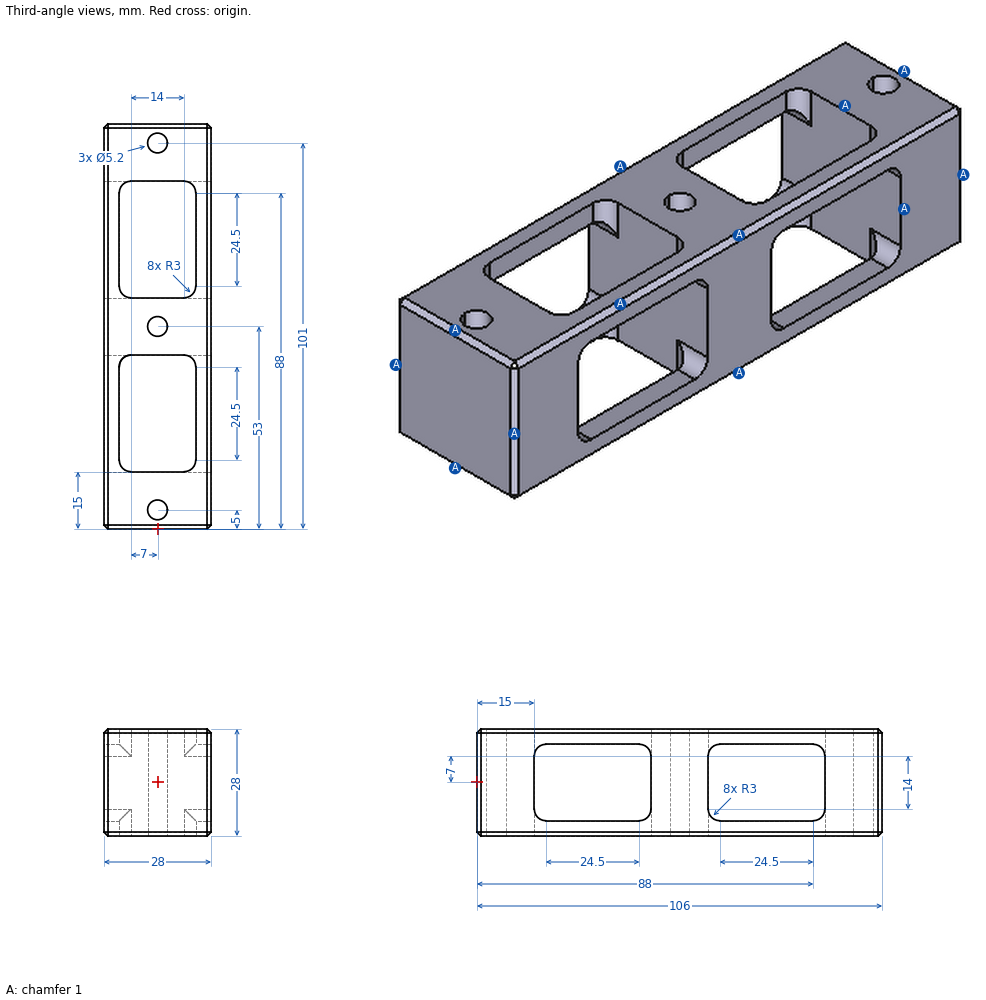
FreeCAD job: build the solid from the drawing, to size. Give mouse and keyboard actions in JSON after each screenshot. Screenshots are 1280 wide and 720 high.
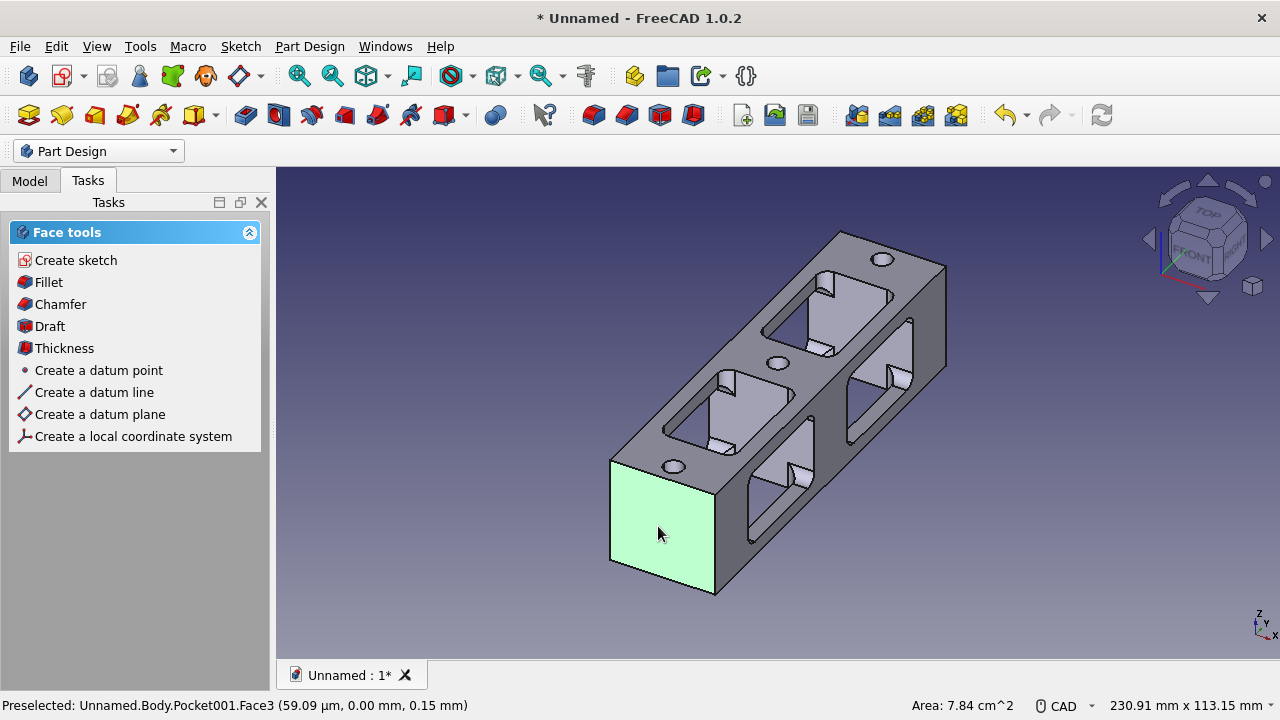
{"action": "left_click", "coordinate": [831, 380], "text": "ctrl"}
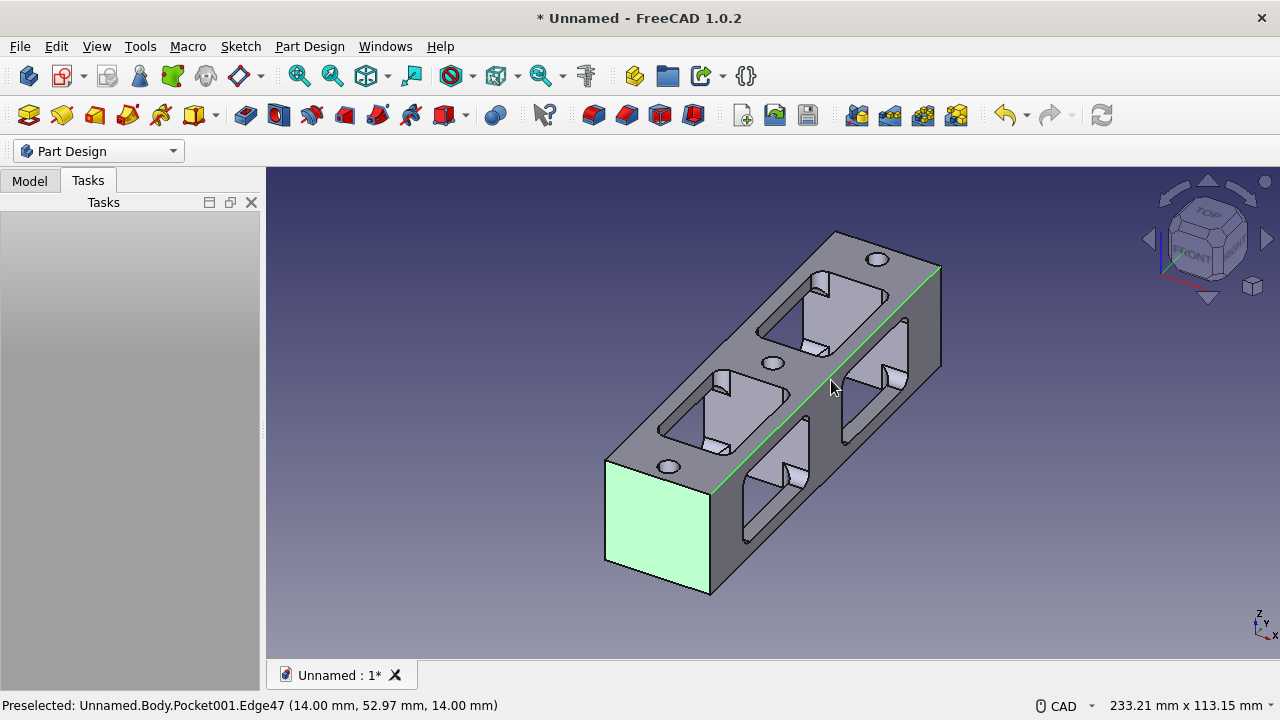
{"action": "key", "text": "0"}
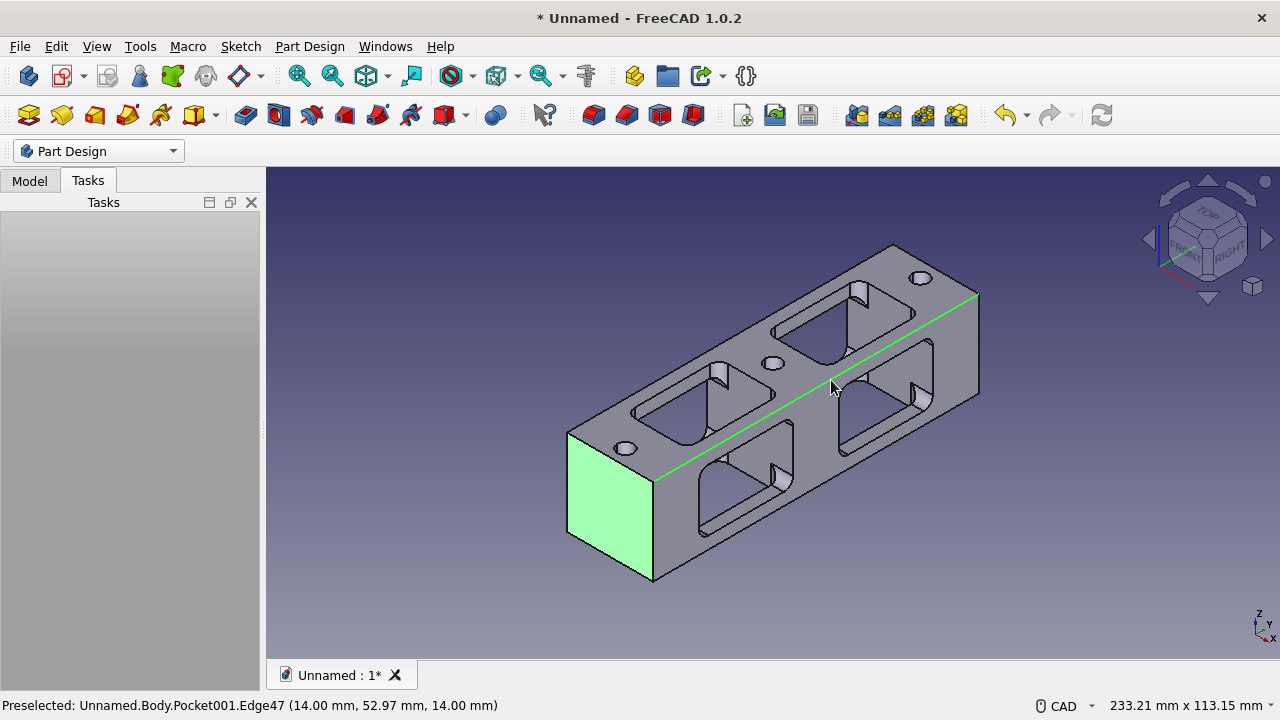
{"action": "key", "text": "2"}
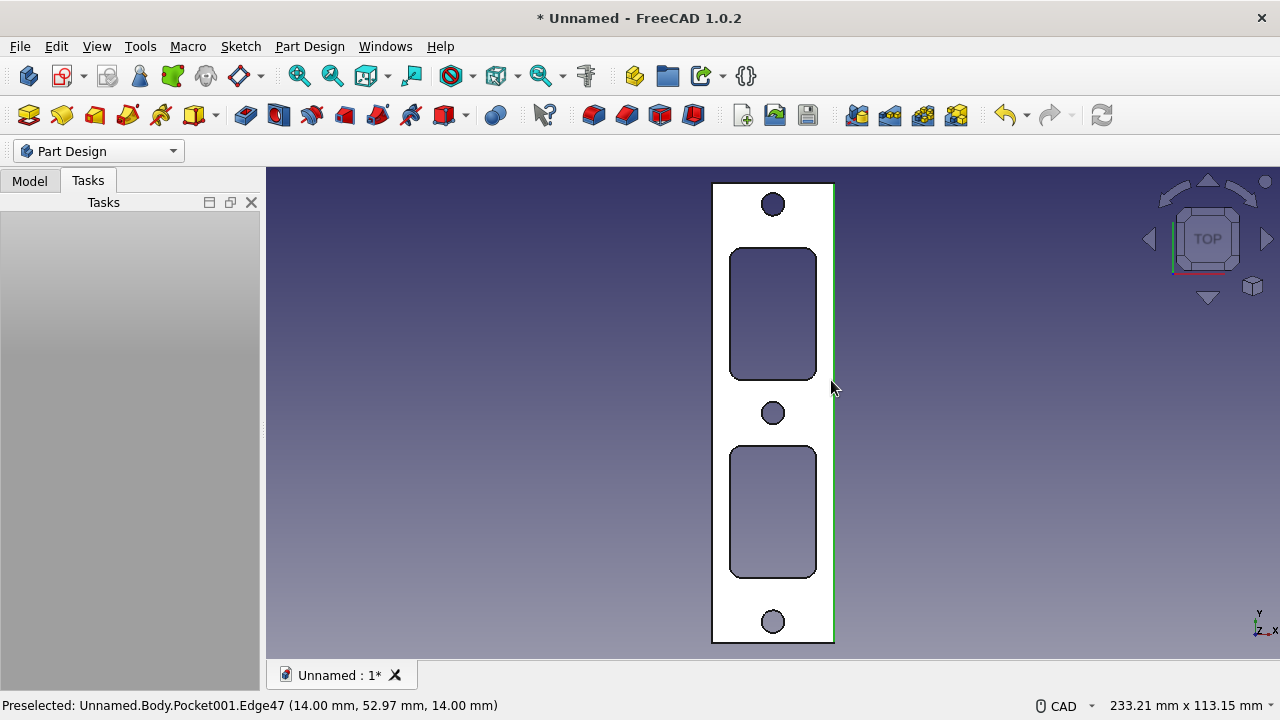
{"action": "left_click", "coordinate": [712, 412], "text": "ctrl"}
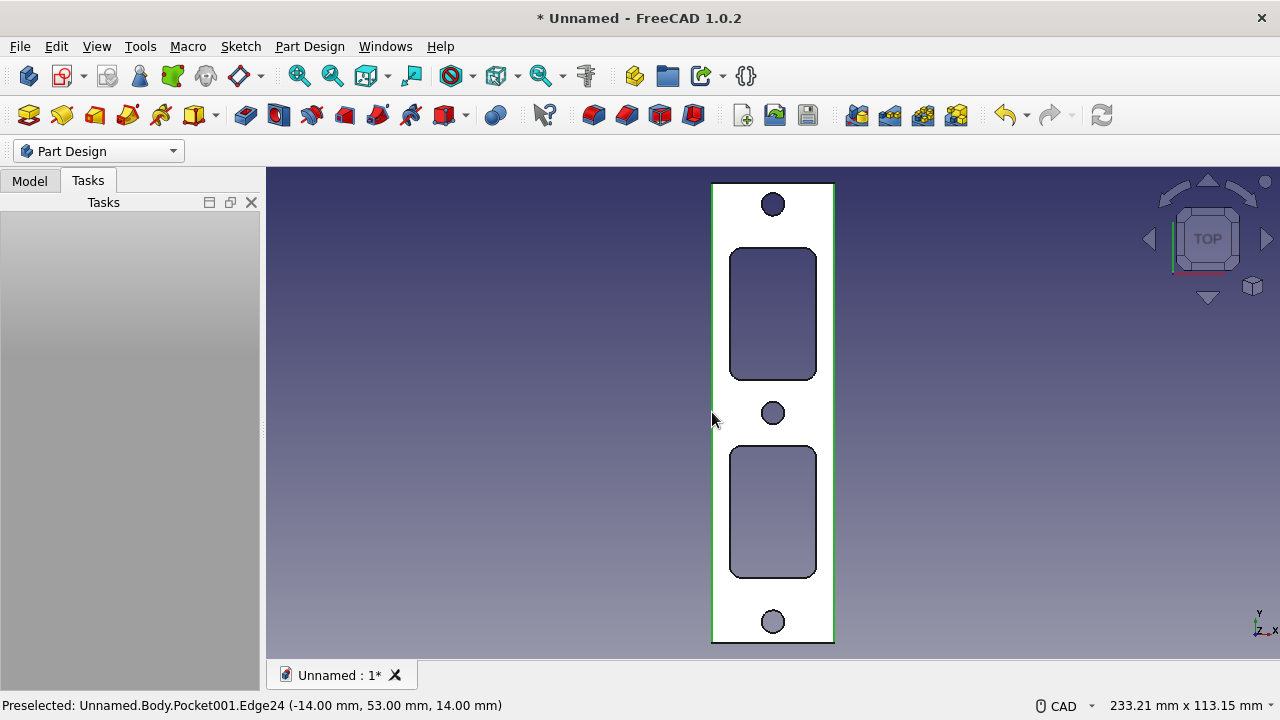
{"action": "key", "text": "1"}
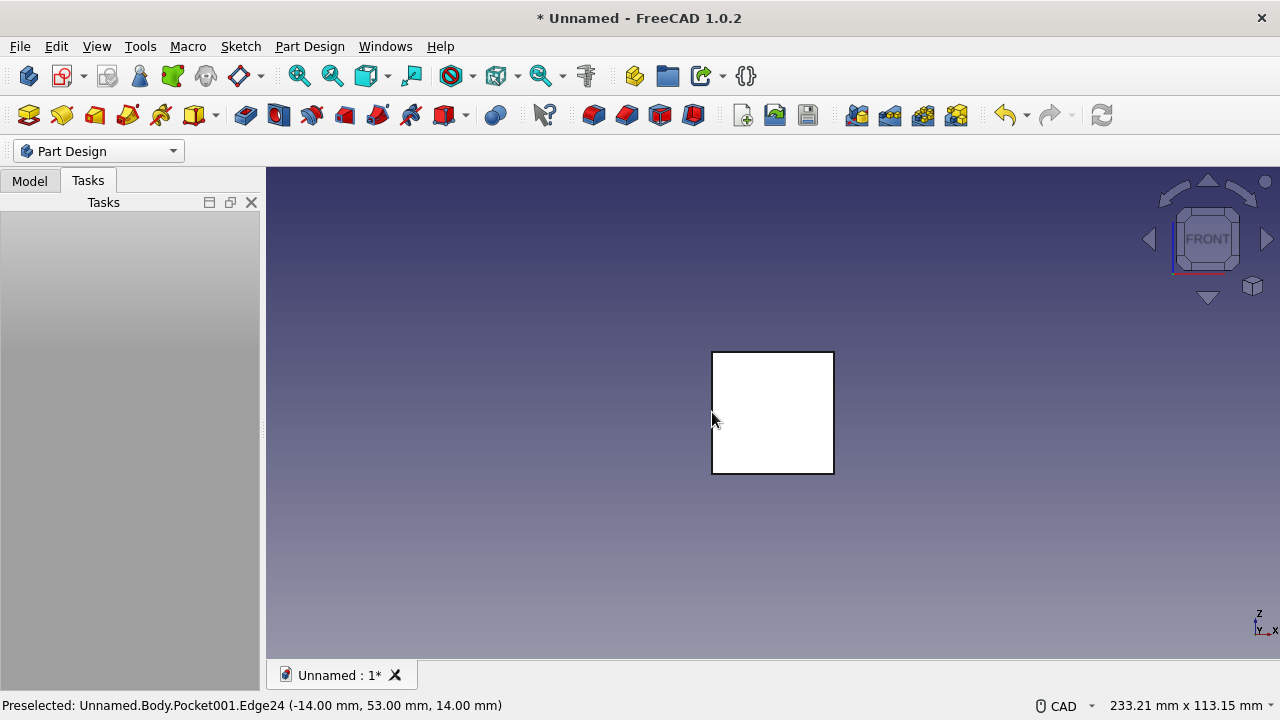
{"action": "left_click", "coordinate": [300, 76]}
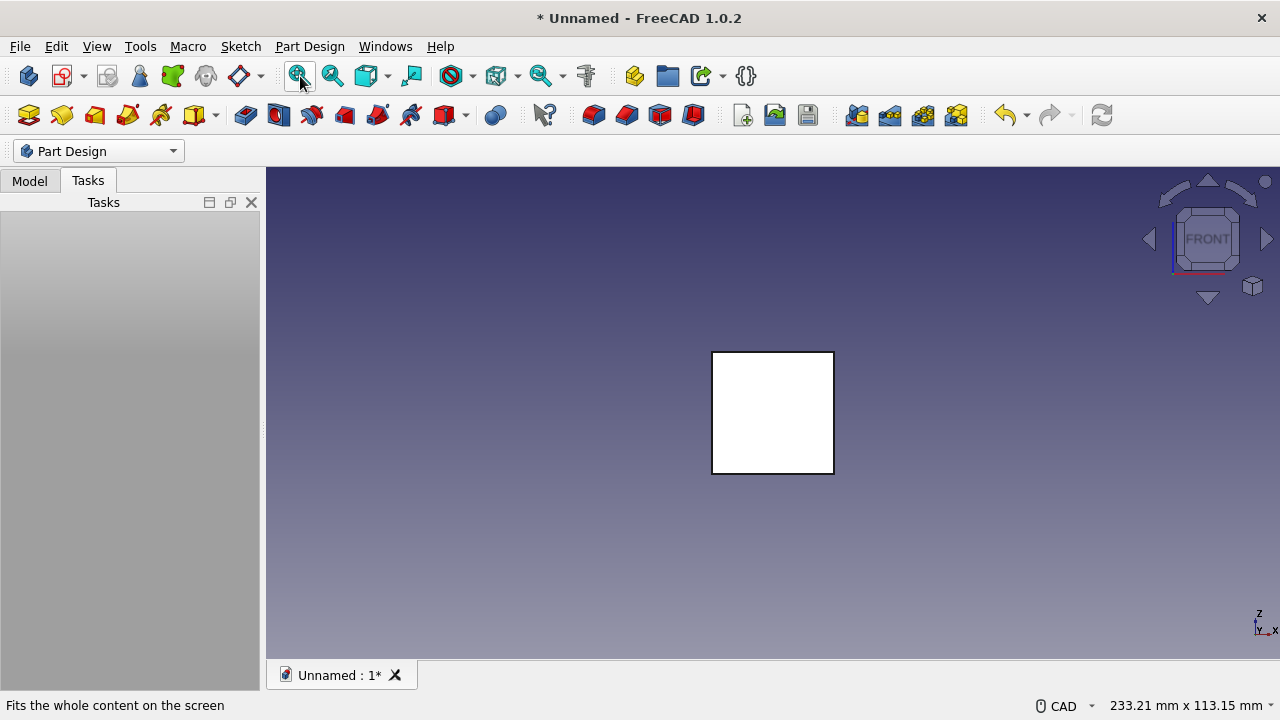
{"action": "key", "text": "3"}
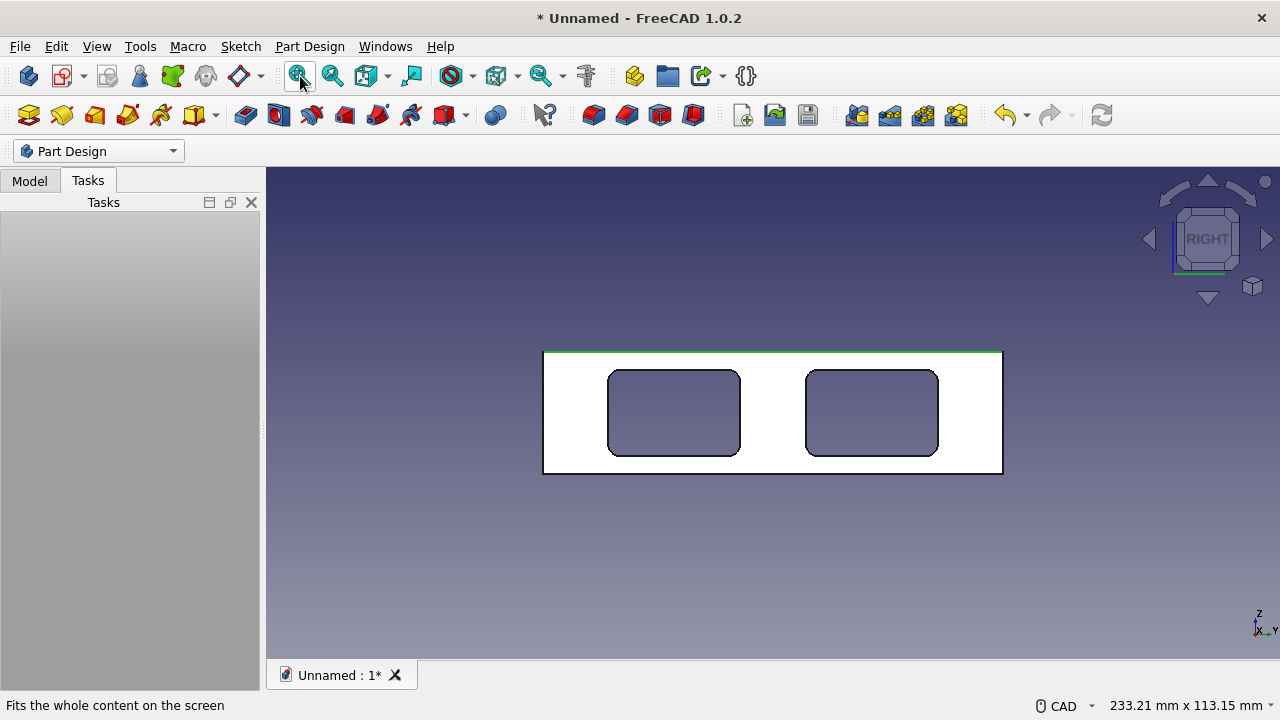
{"action": "left_click", "coordinate": [773, 473], "text": "ctrl"}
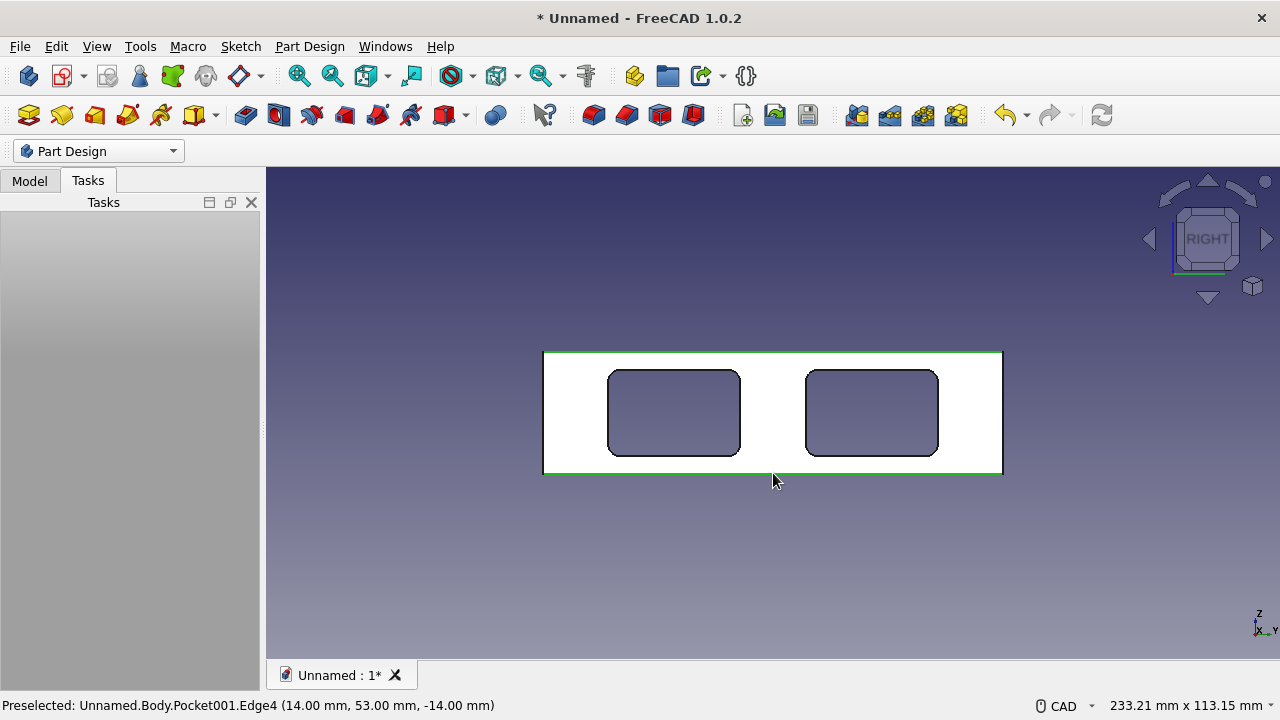
{"action": "key", "text": "5"}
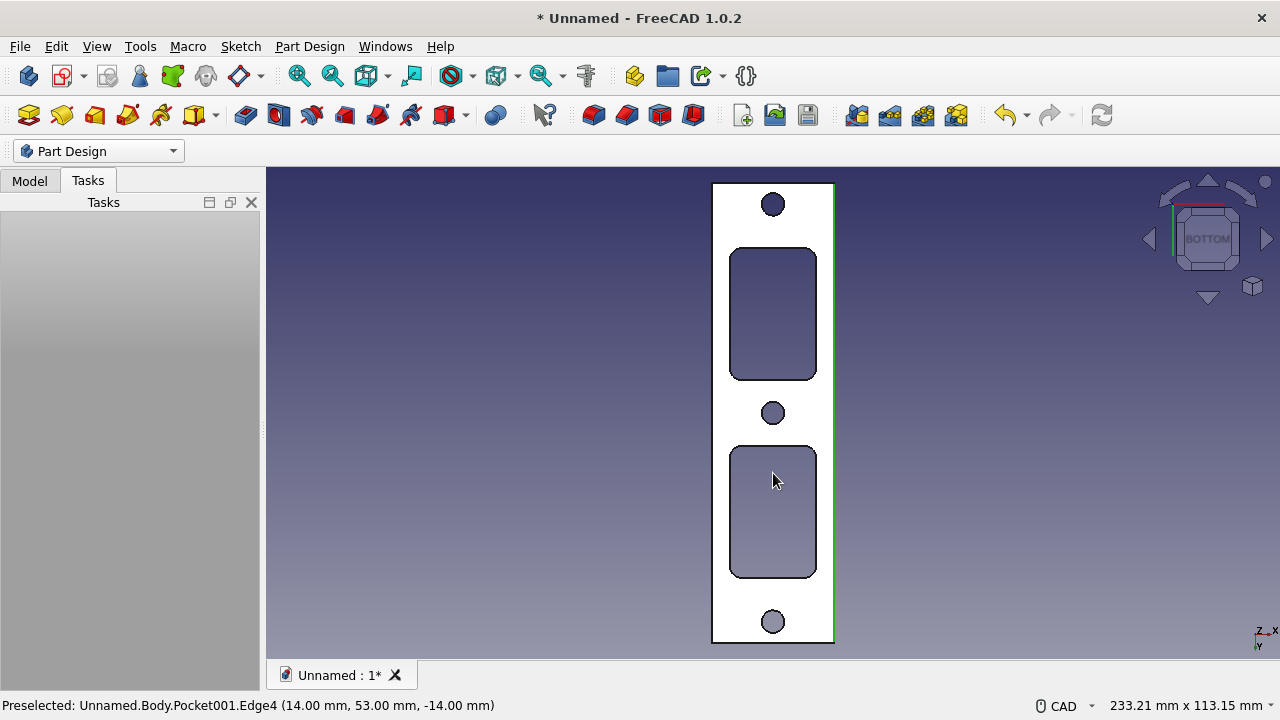
{"action": "left_click", "coordinate": [712, 412], "text": "ctrl"}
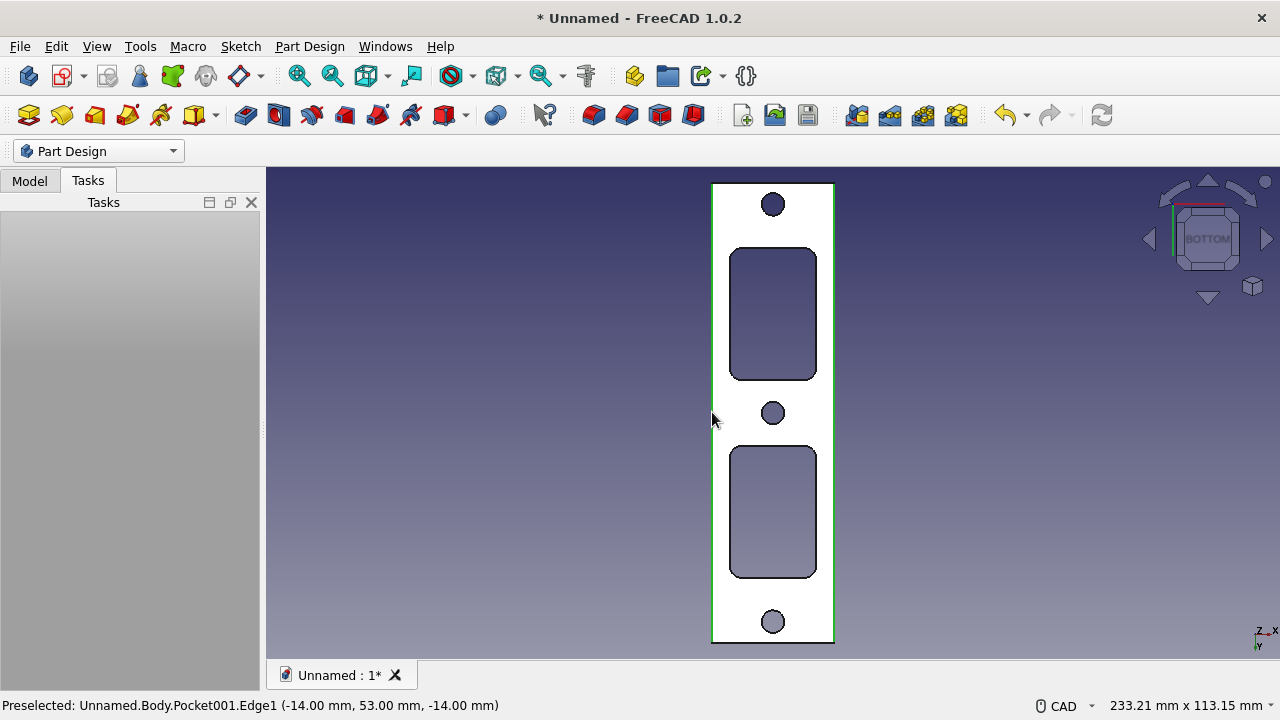
{"action": "key", "text": "4"}